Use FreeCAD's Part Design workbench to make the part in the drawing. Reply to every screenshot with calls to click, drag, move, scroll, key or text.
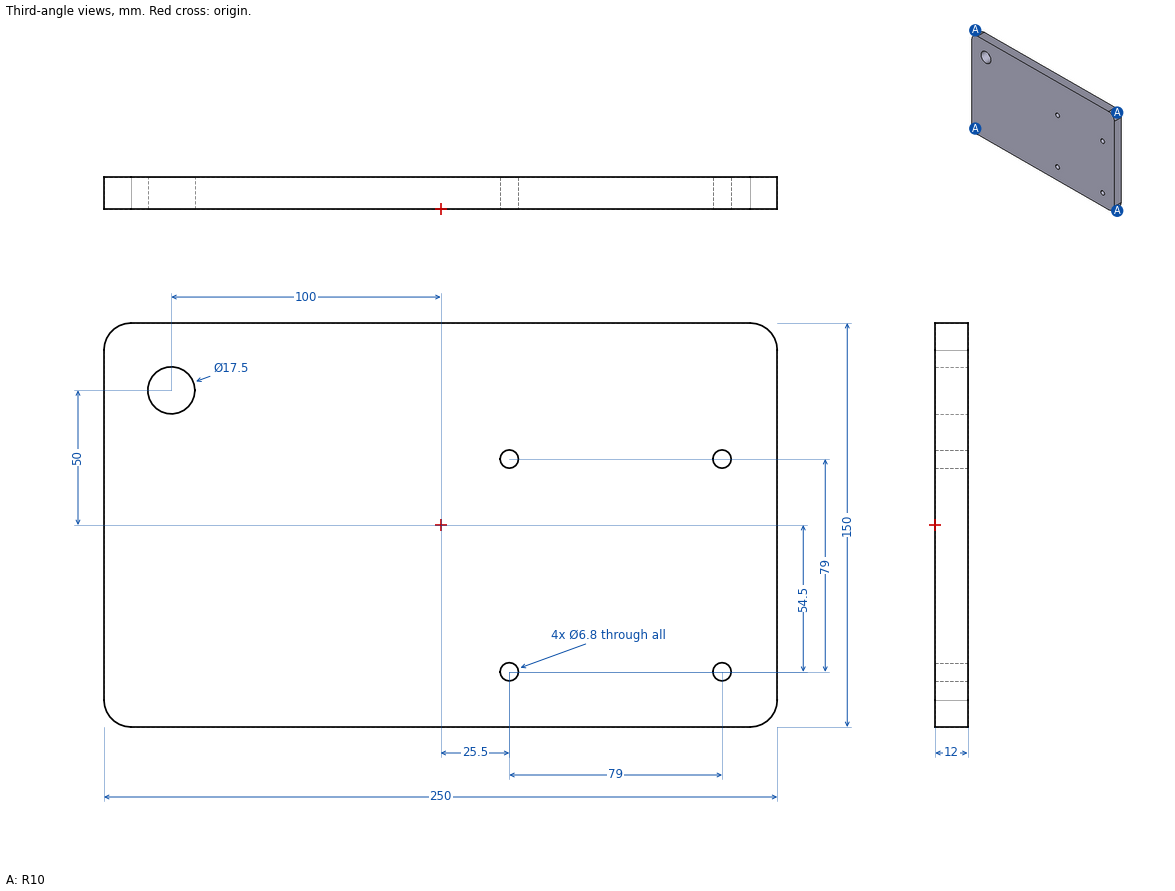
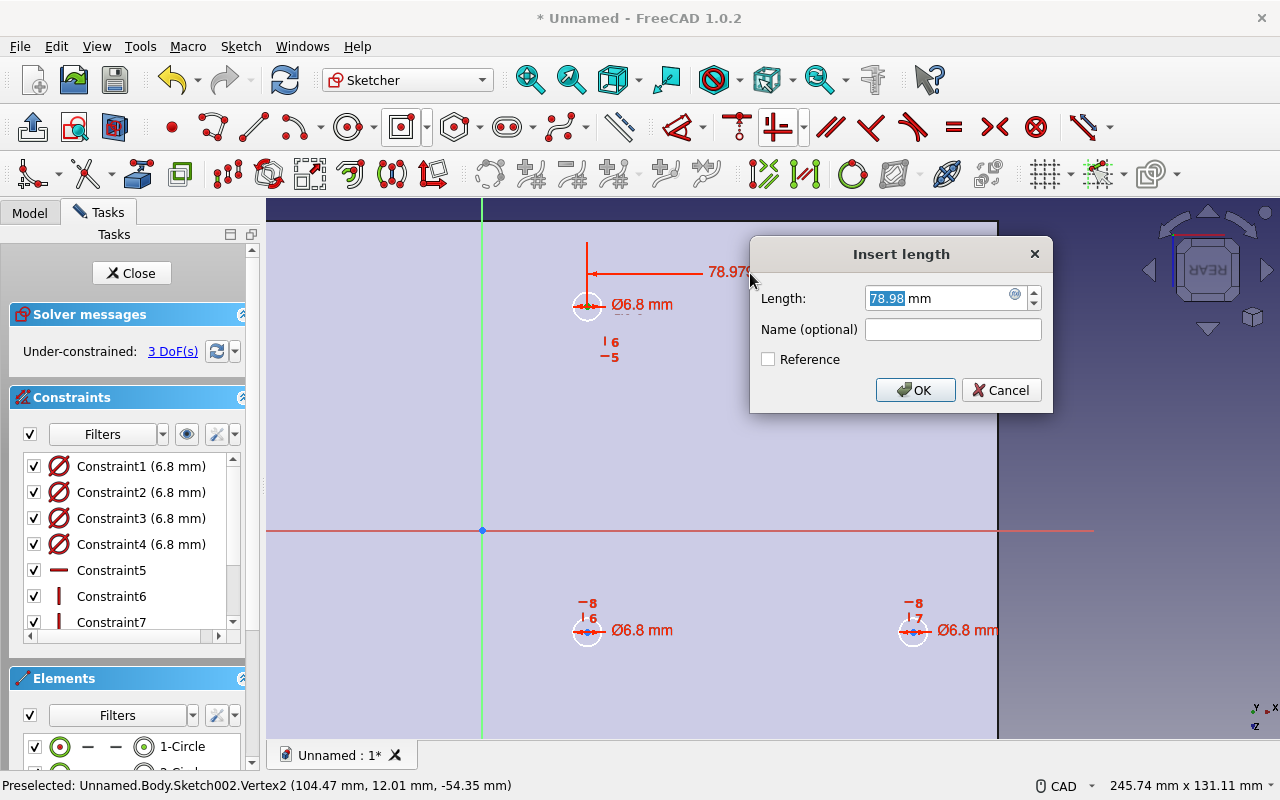
text(79)
key(Return)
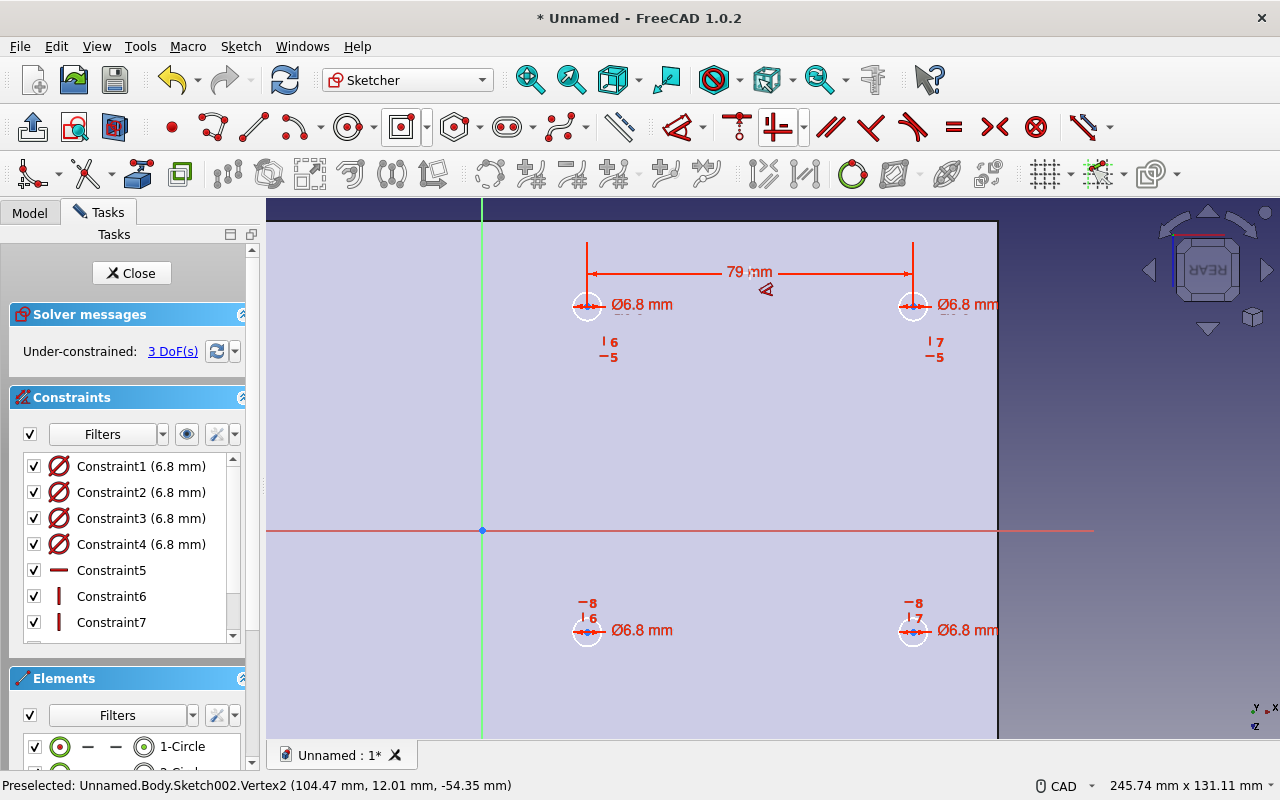
click(587, 307)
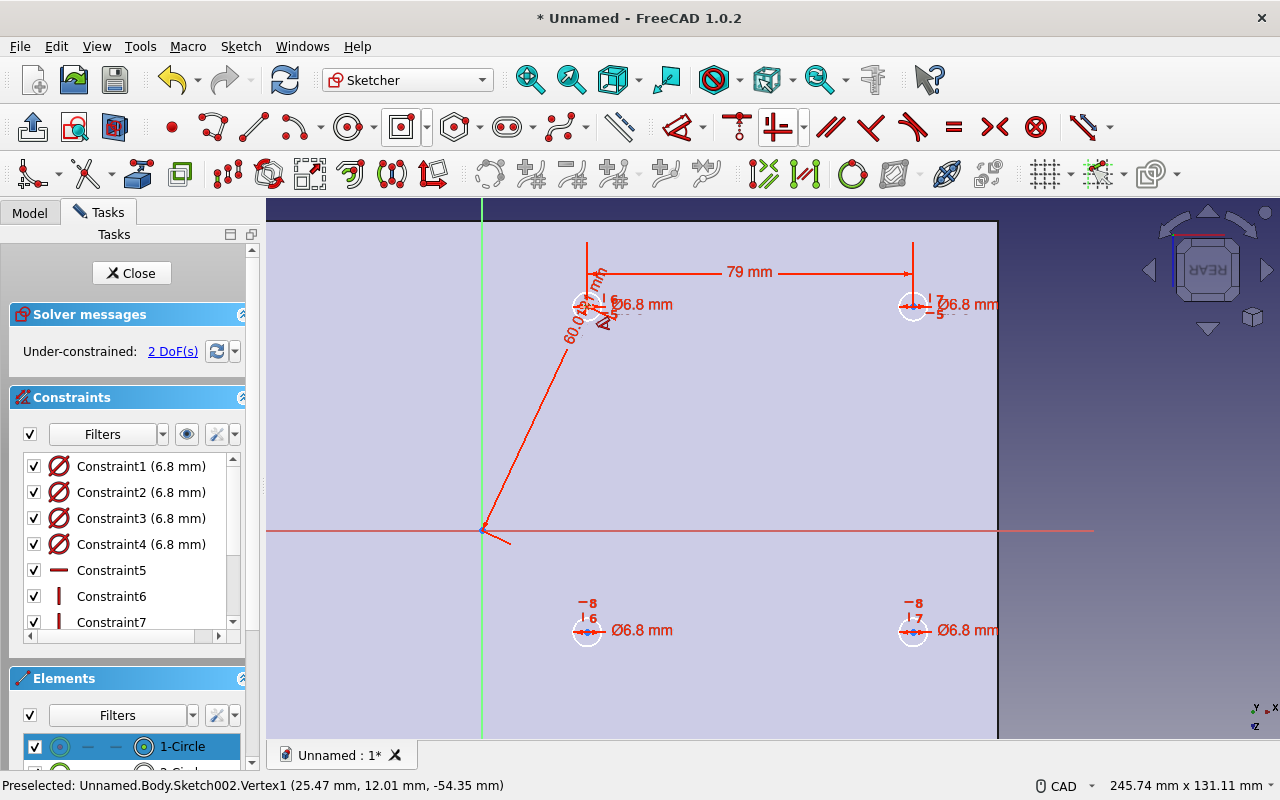
click(587, 632)
click(553, 469)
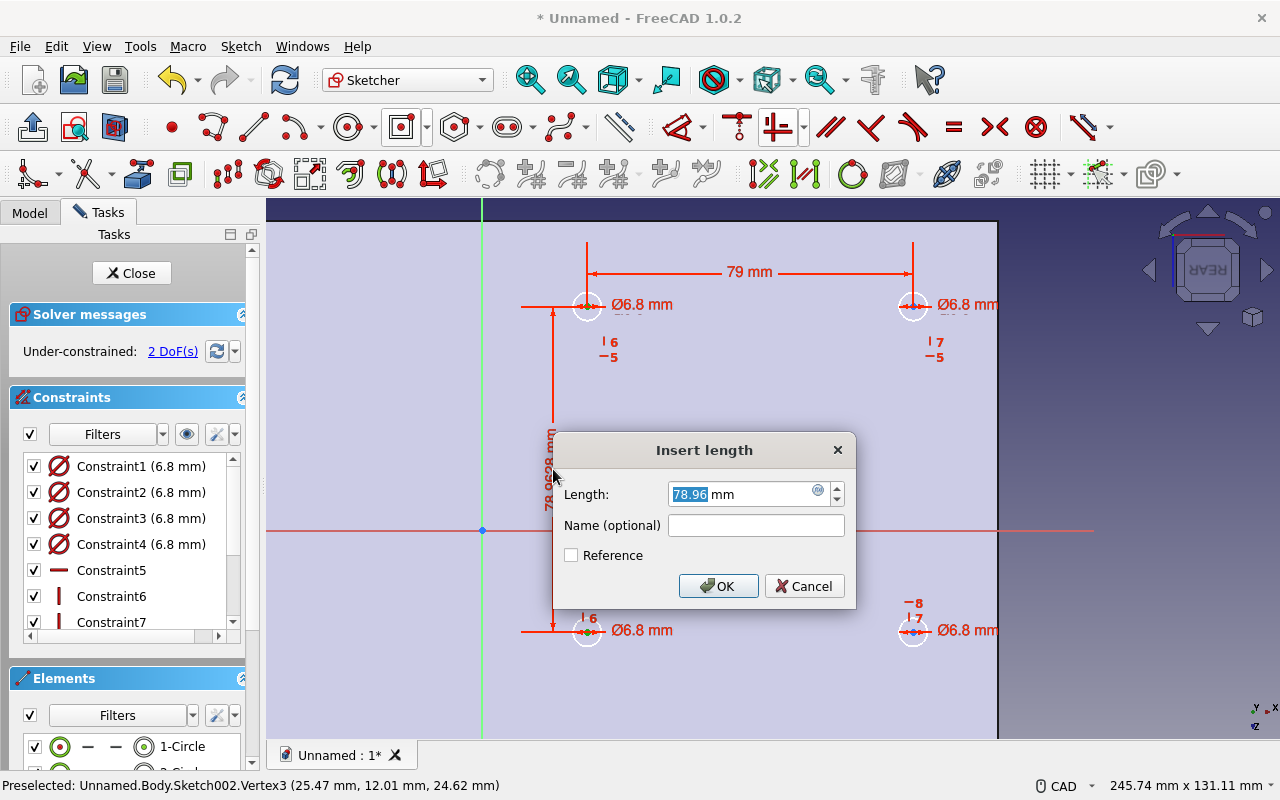
text(79)
key(Return)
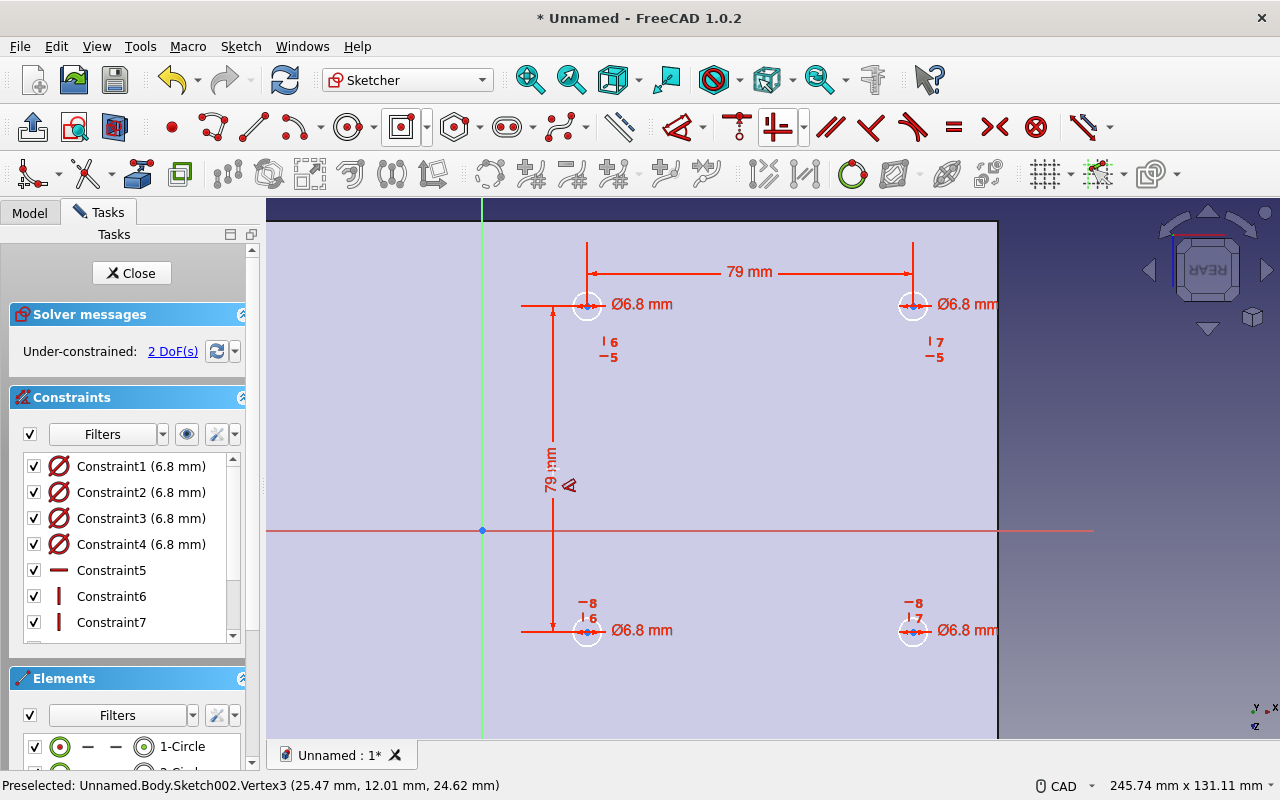
click(587, 306)
click(535, 272)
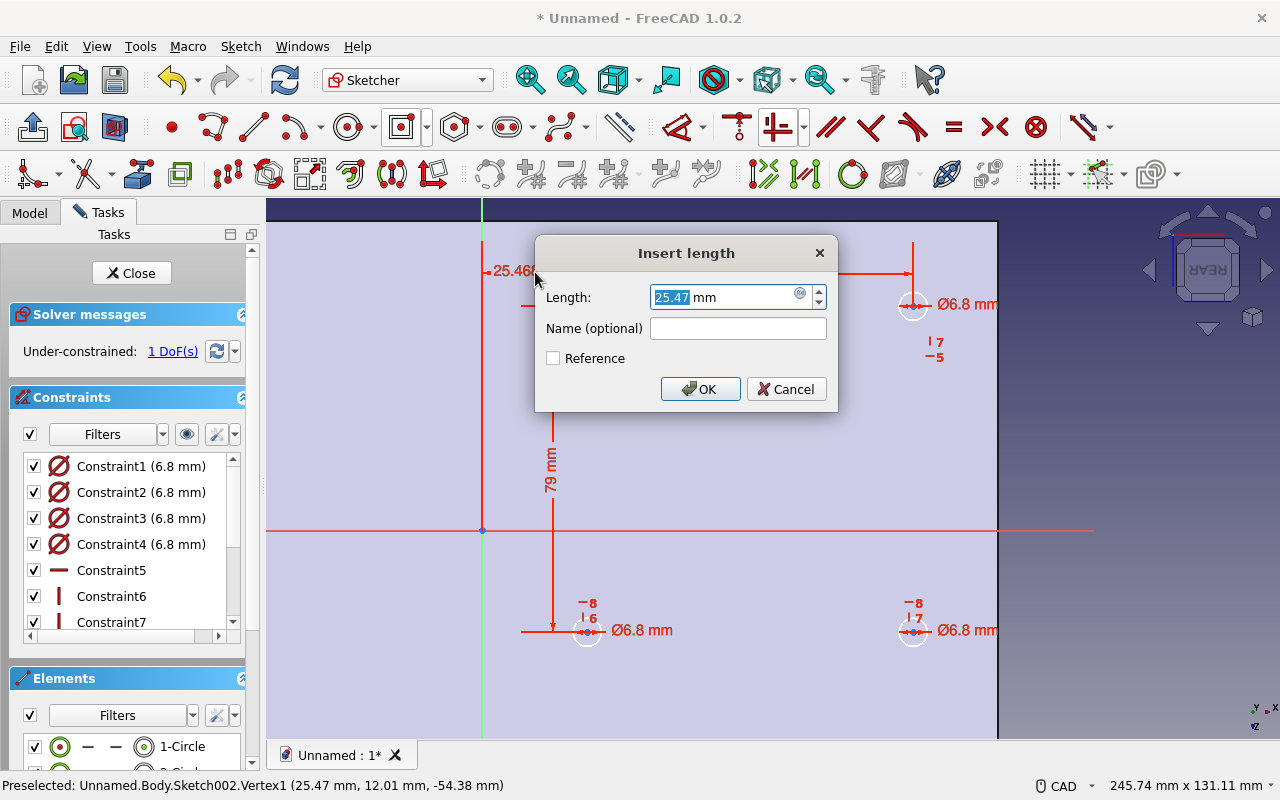
text(25.5)
key(Return)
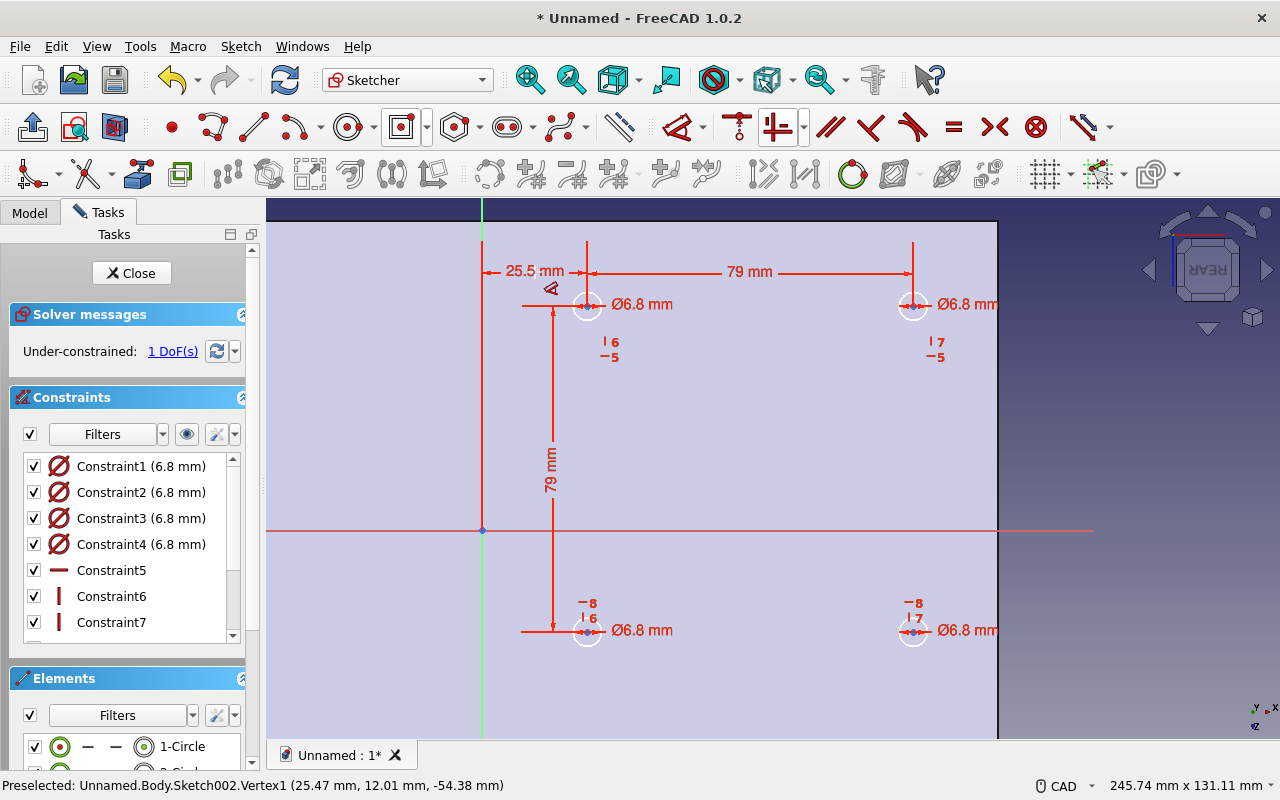
click(587, 306)
click(448, 419)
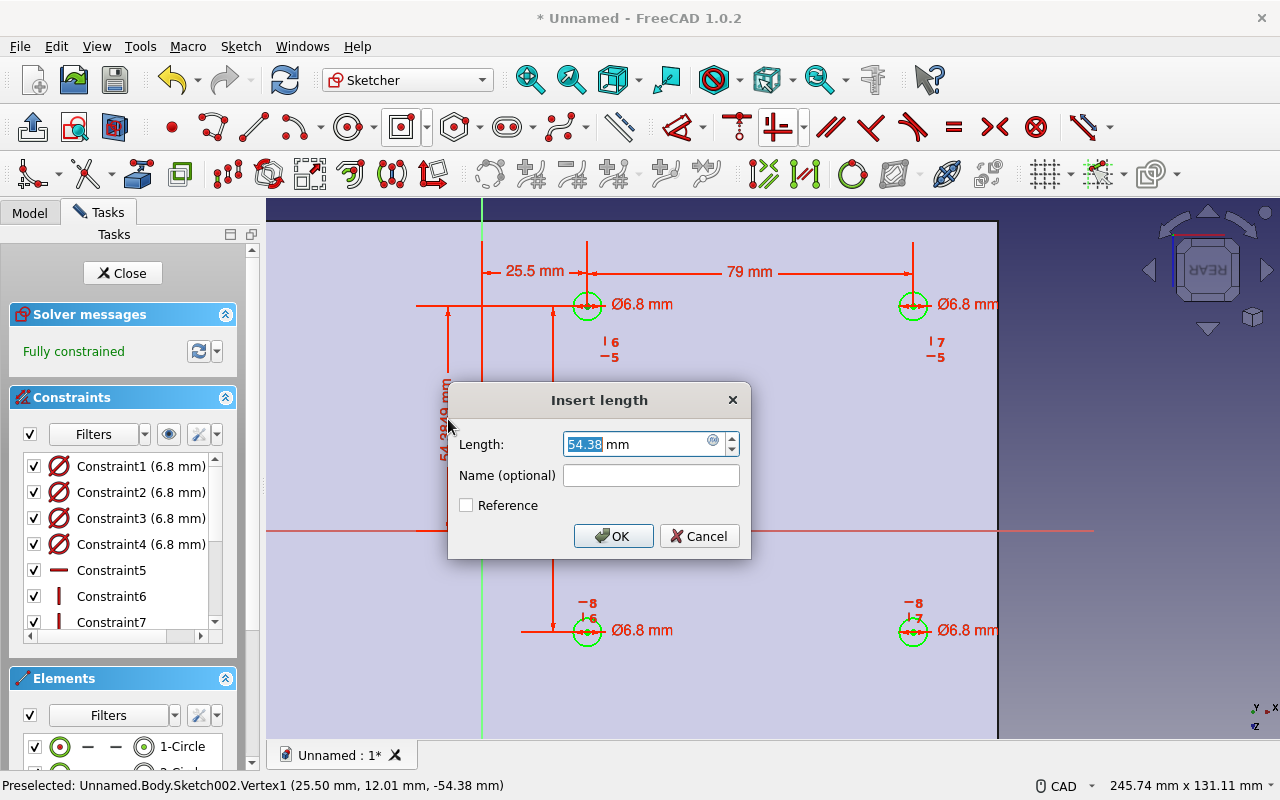
text(54.5)
key(Return)
key(Escape)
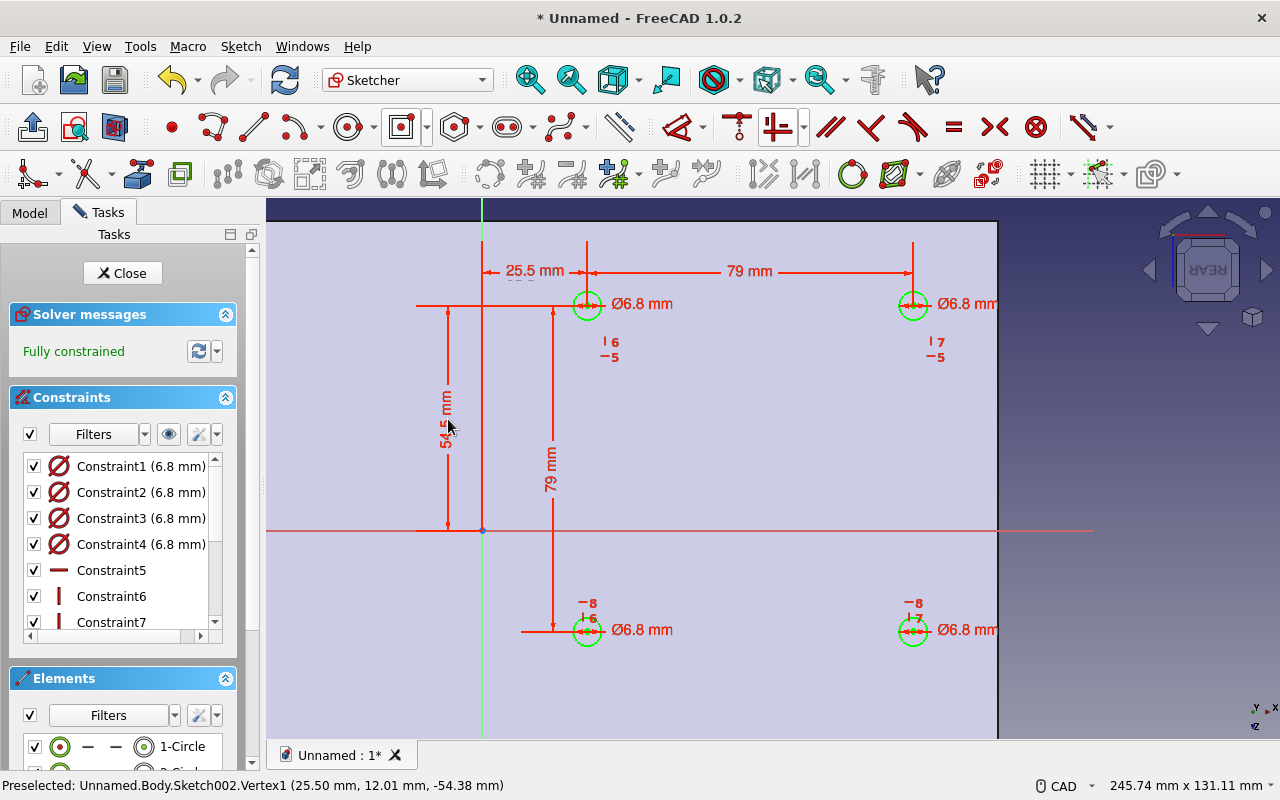
click(123, 273)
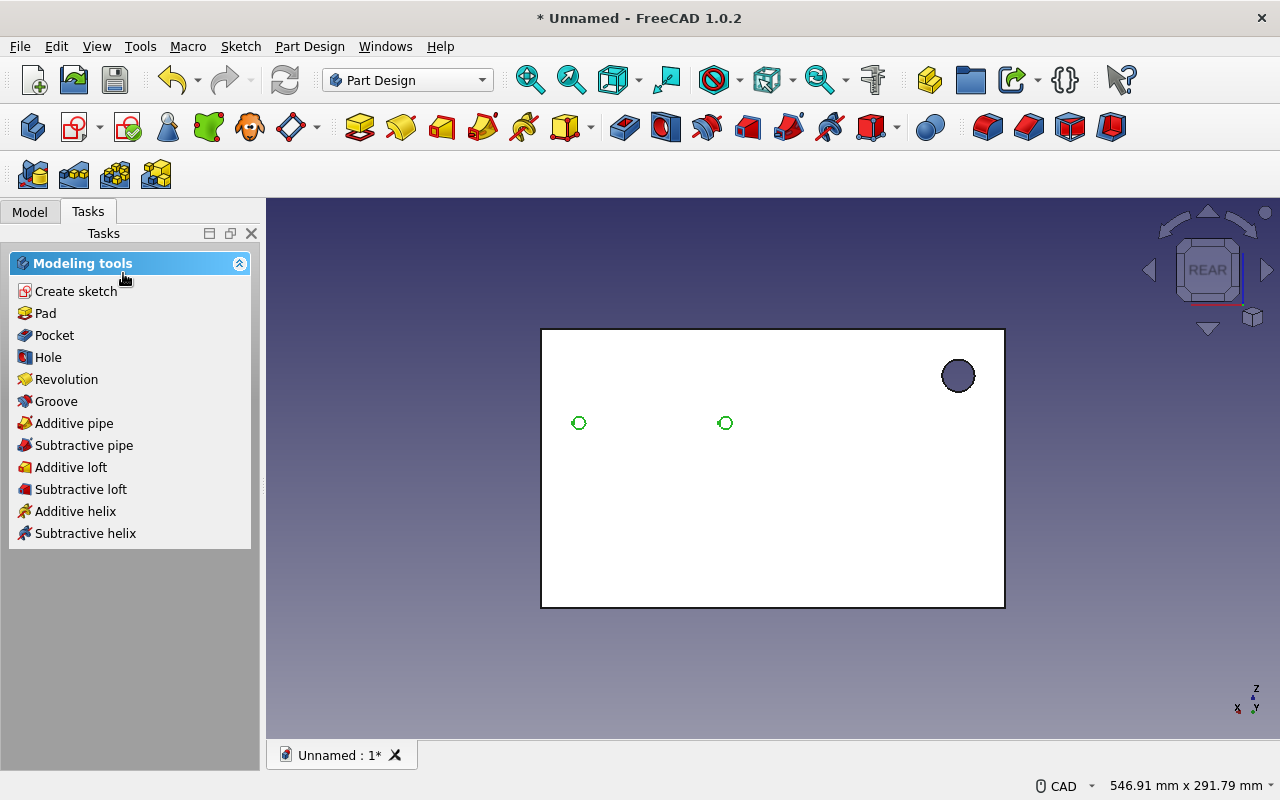
click(666, 128)